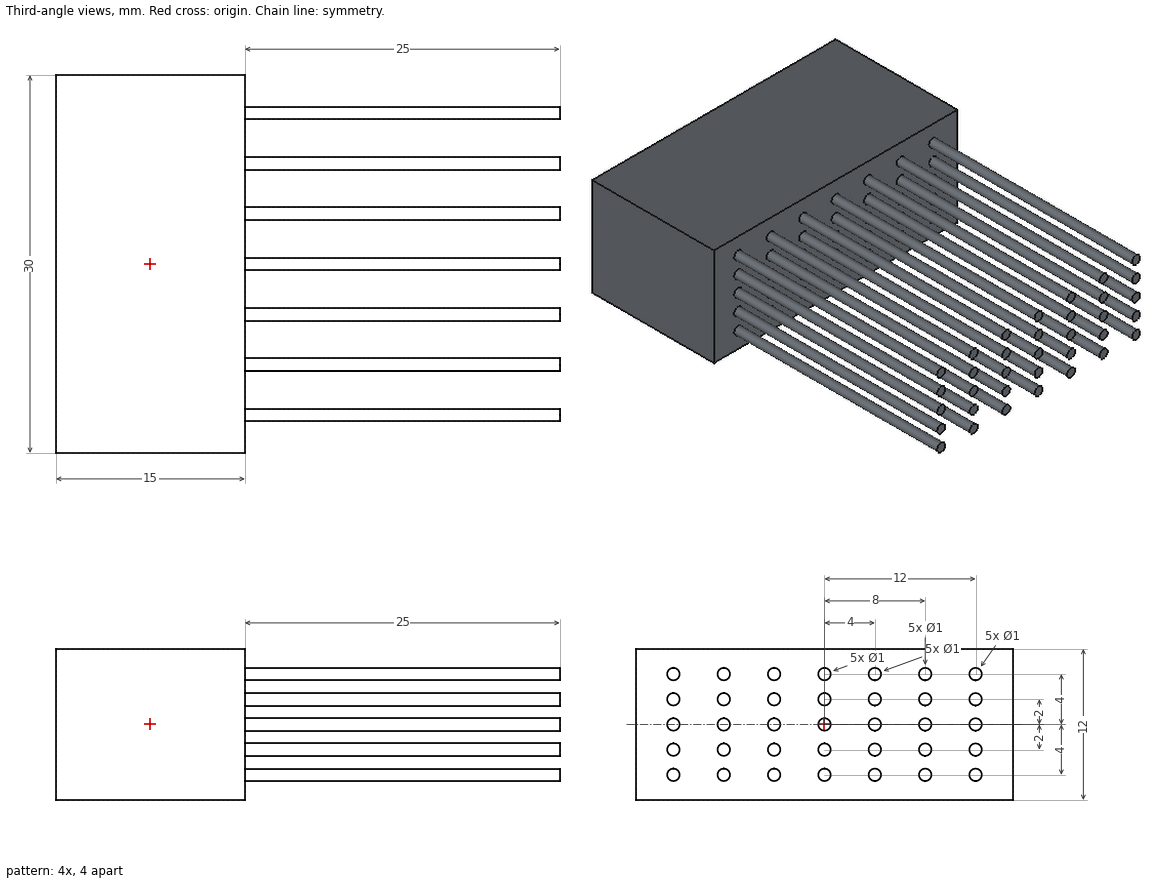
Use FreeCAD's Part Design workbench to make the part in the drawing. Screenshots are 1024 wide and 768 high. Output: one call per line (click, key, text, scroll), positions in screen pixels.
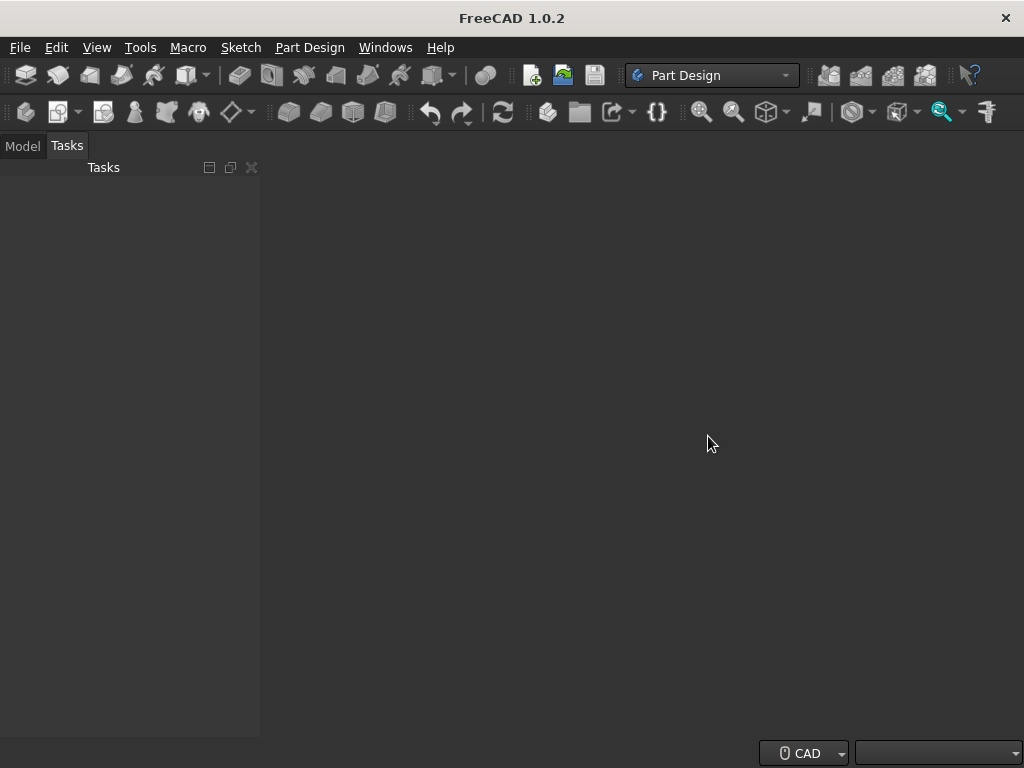
key(ctrl+n)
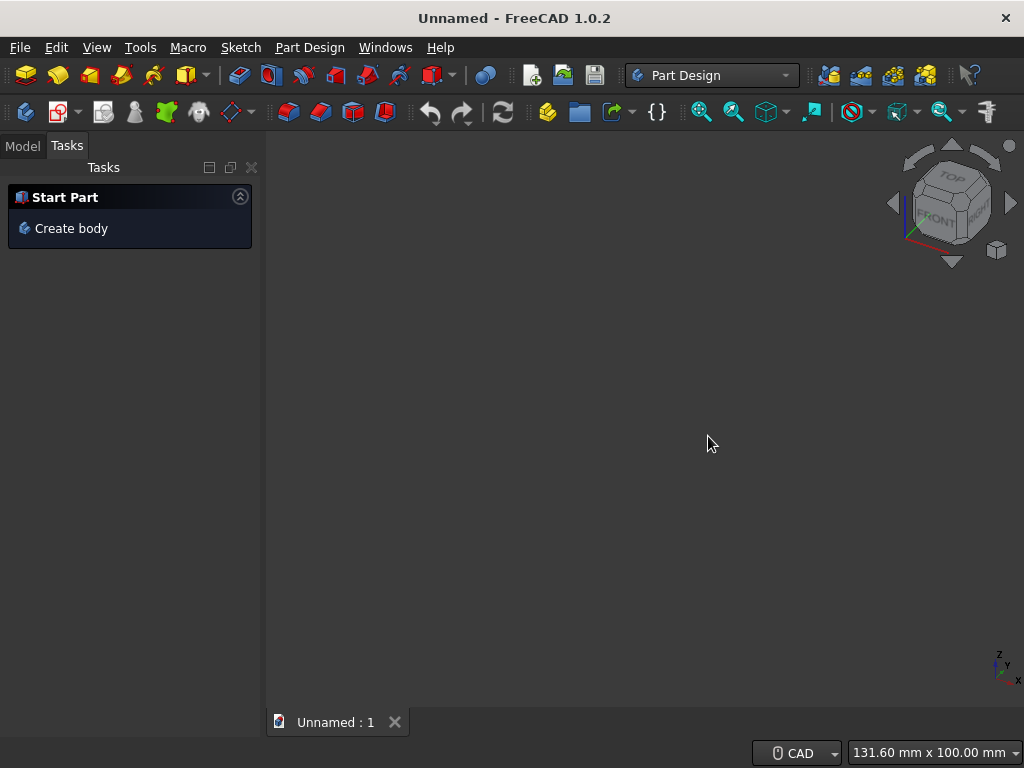
click(58, 112)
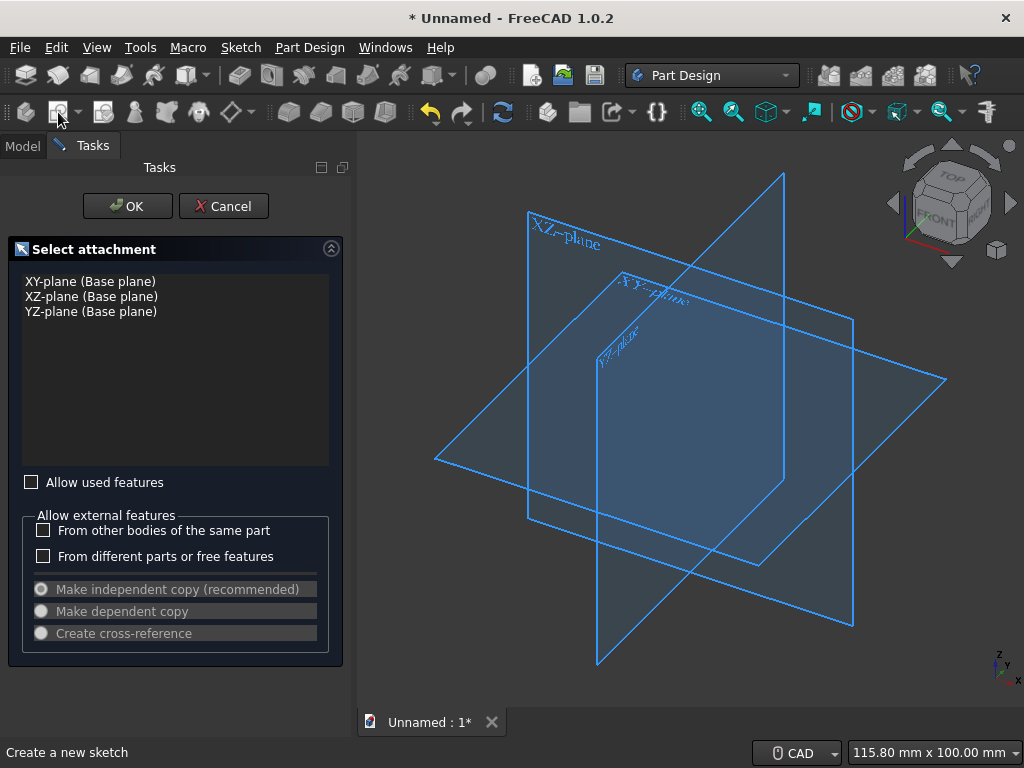
click(82, 282)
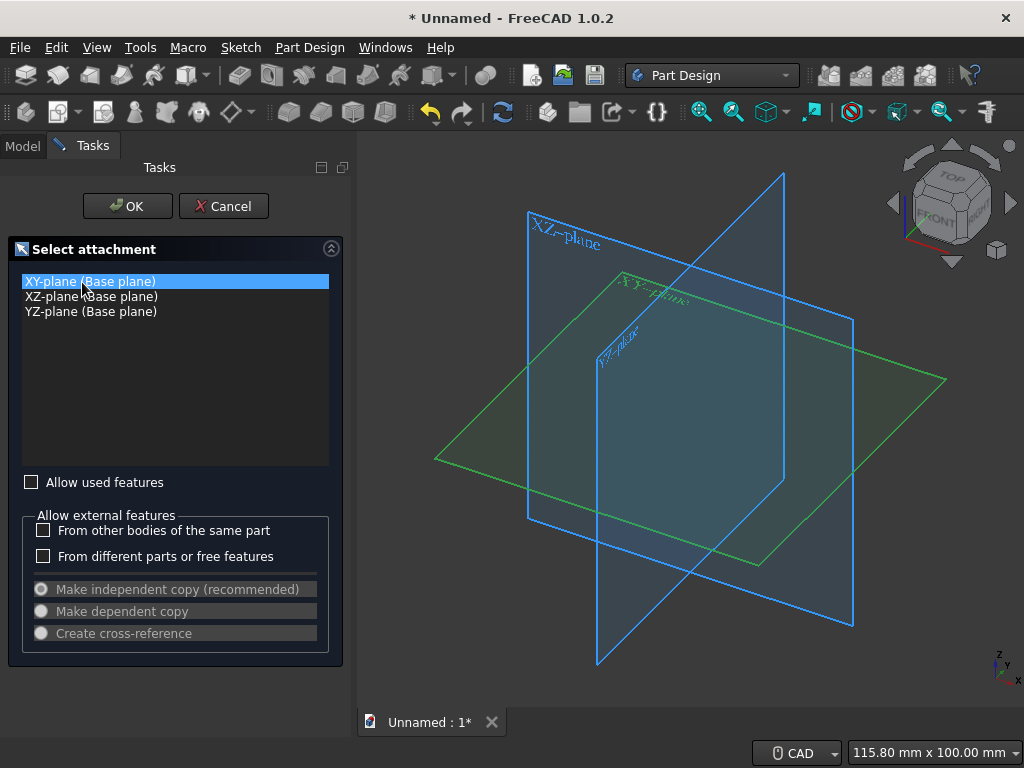
click(128, 206)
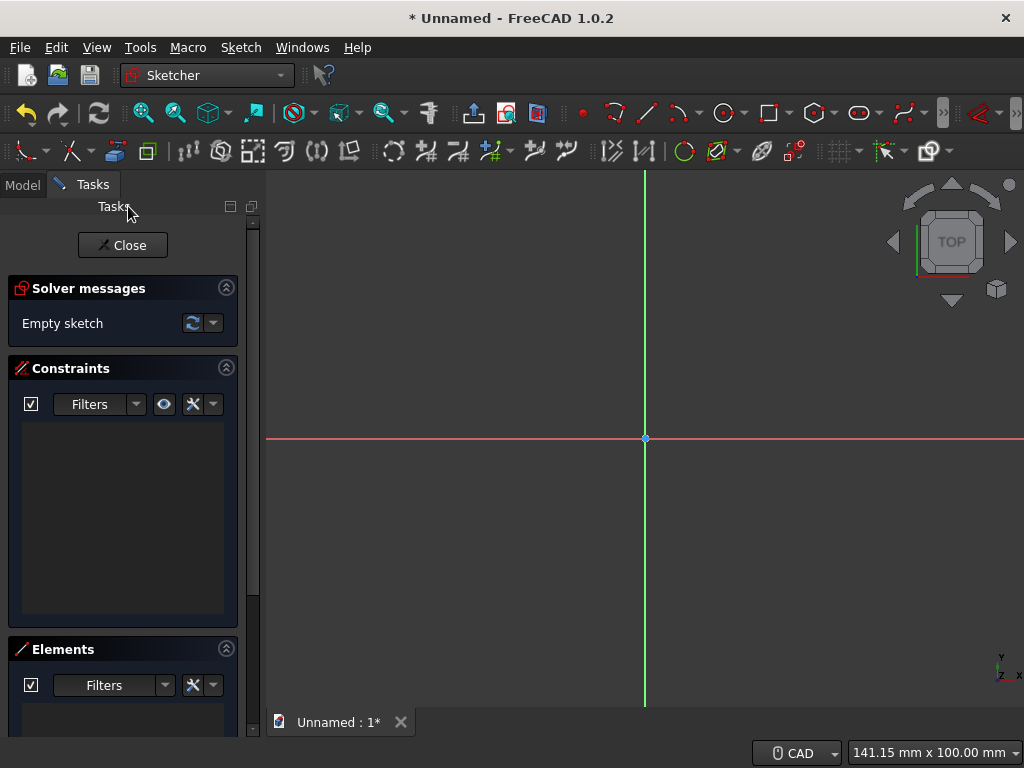
scroll(701, 438, up, 4)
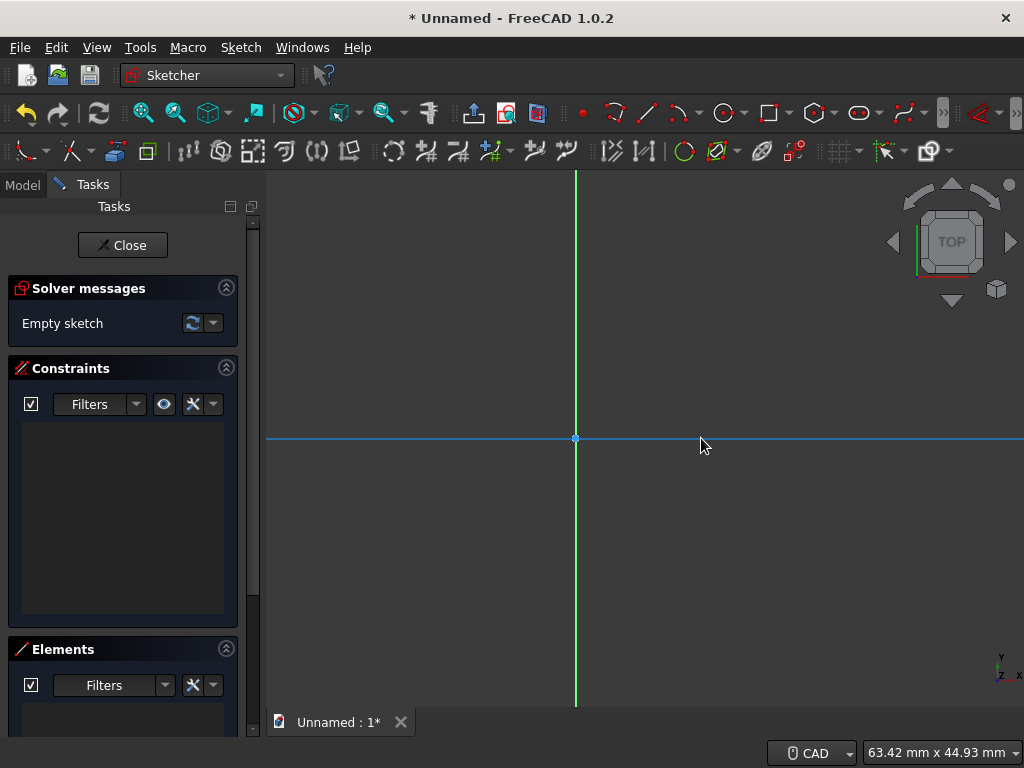
key(g)
key(v)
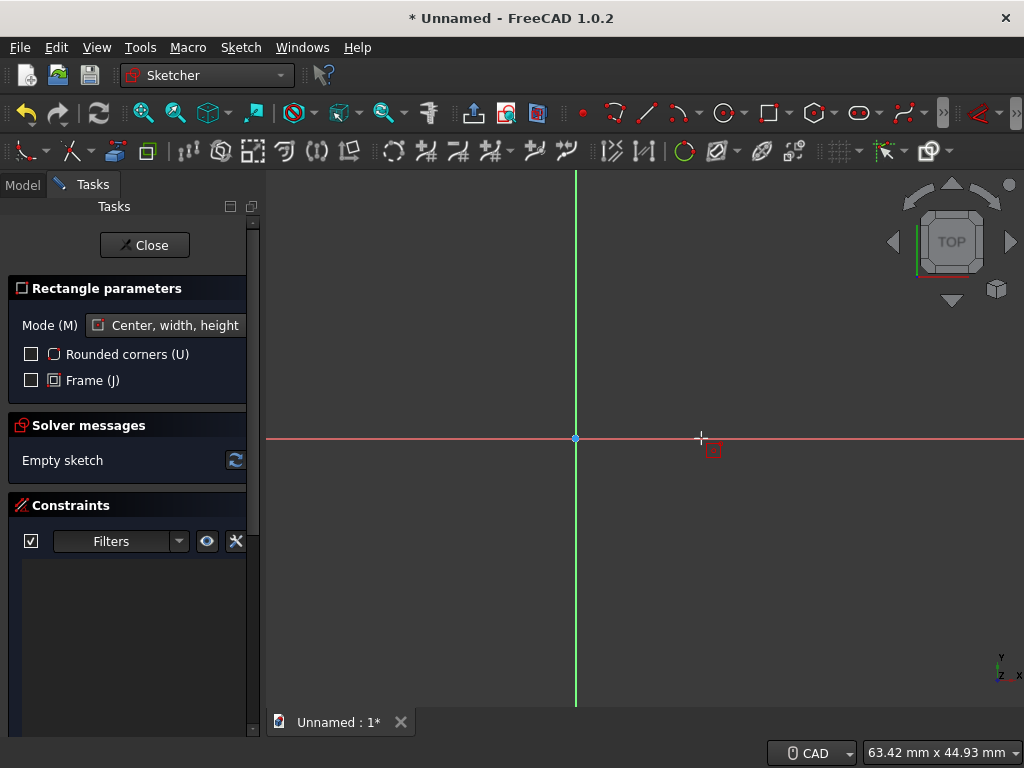
click(576, 438)
move(665, 259)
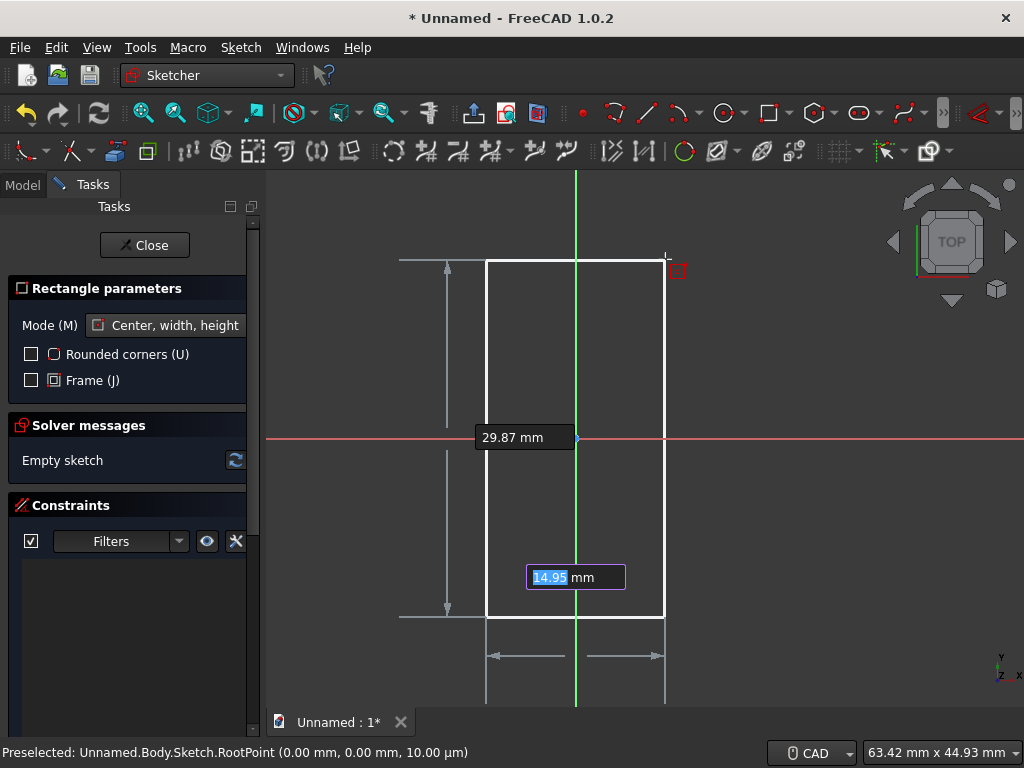
text(15)
key(Tab)
text(30)
key(Return)
key(Escape)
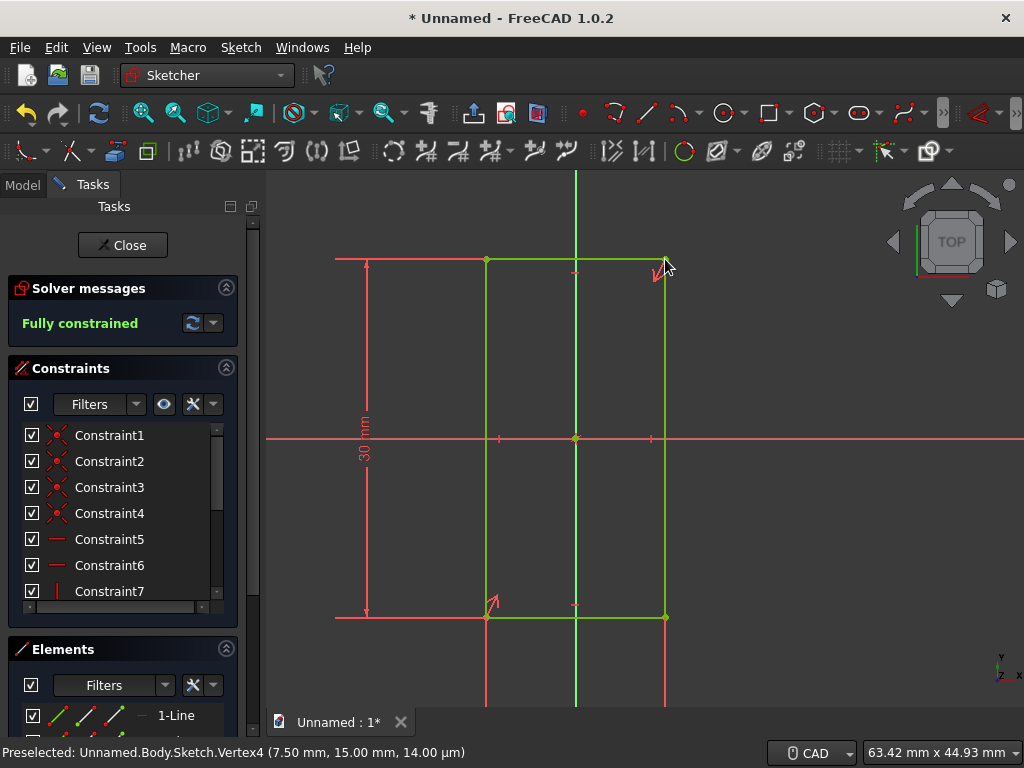
click(123, 245)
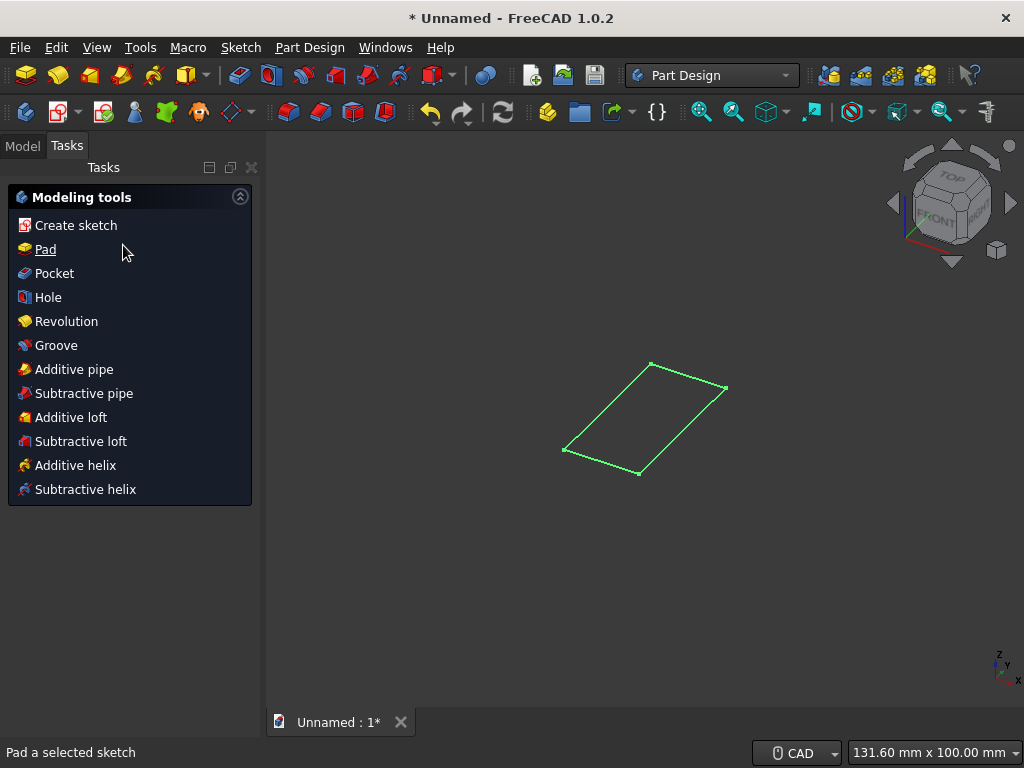
click(26, 76)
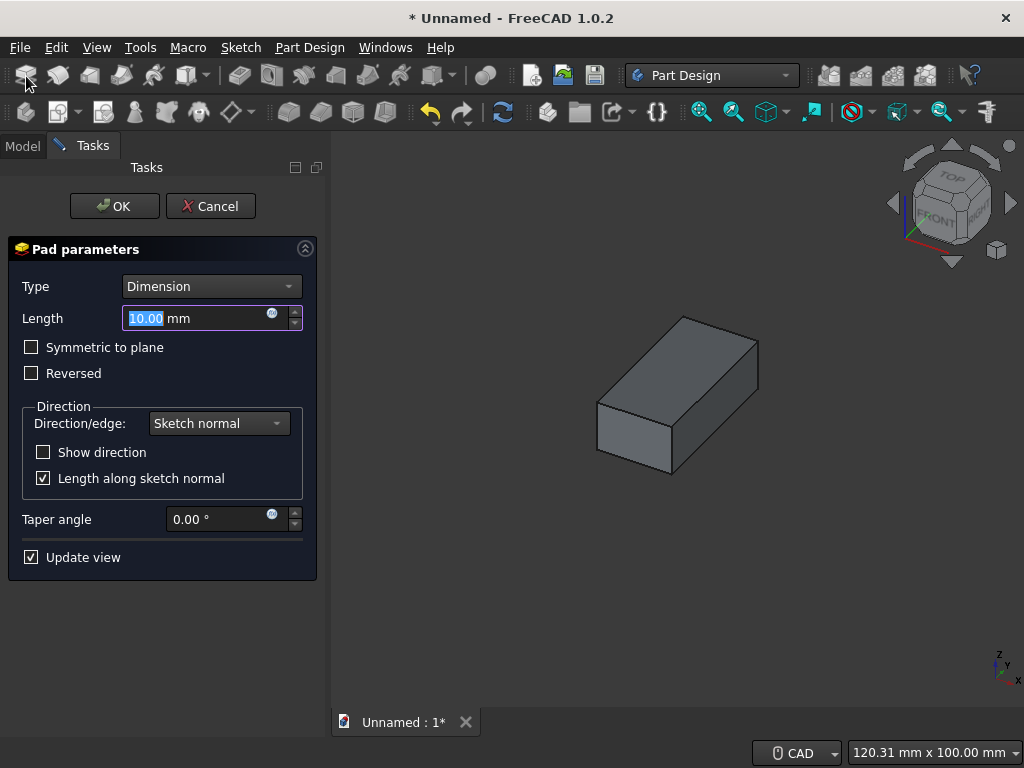
text(12)
key(Tab)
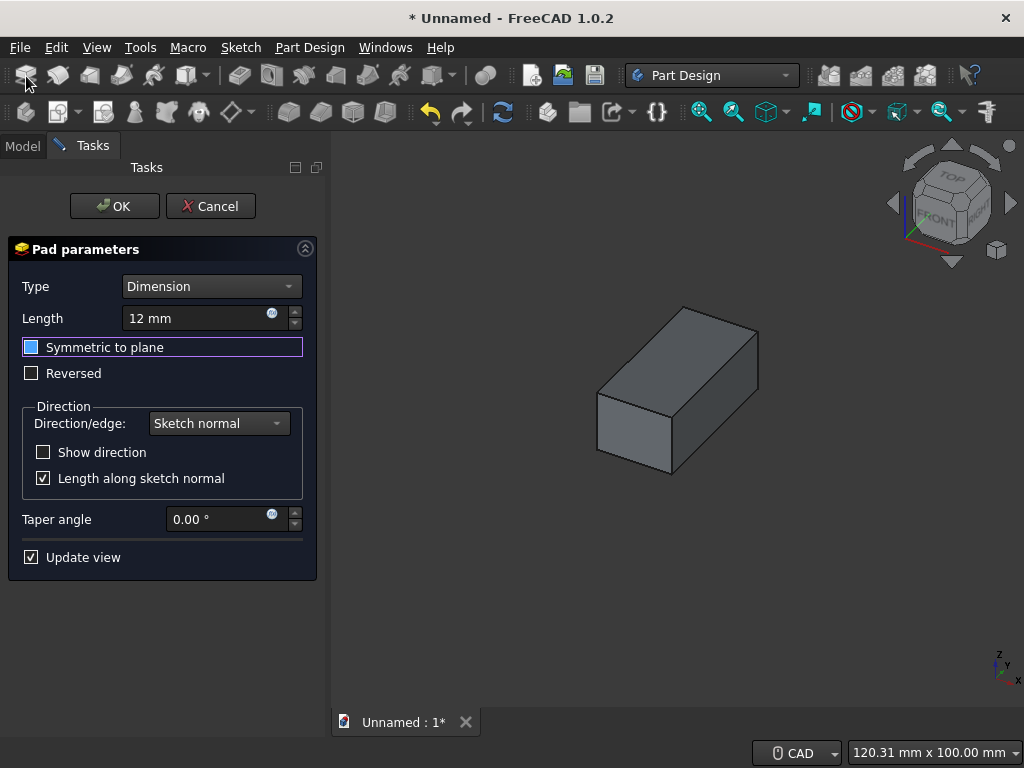
click(30, 347)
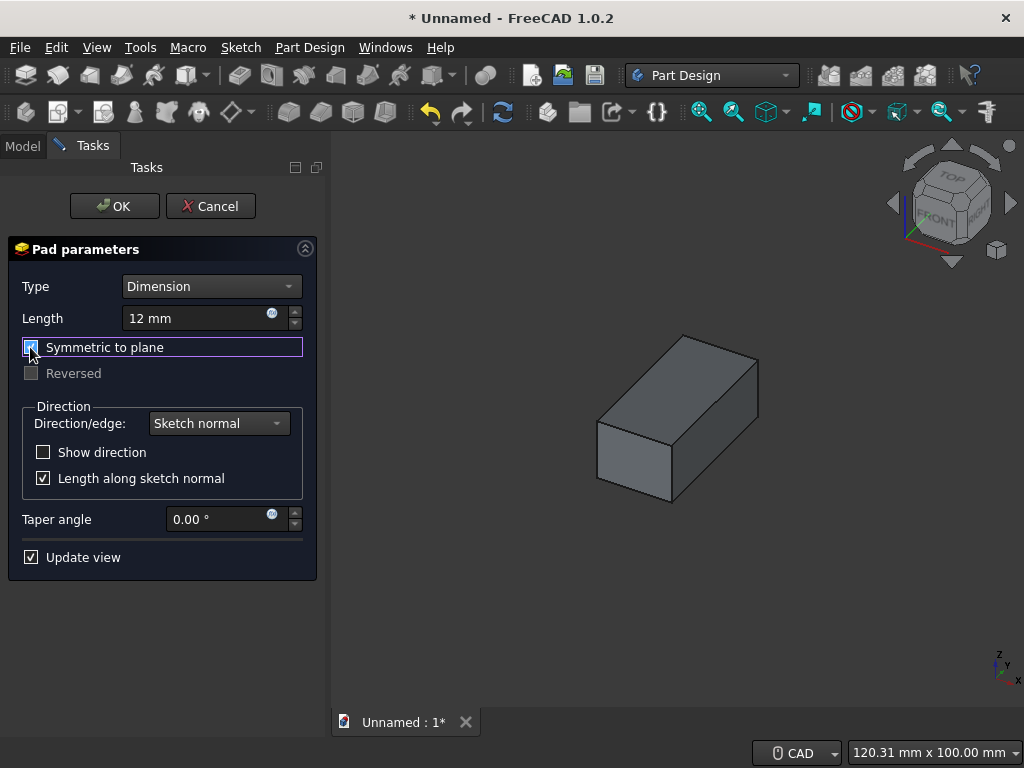
click(115, 206)